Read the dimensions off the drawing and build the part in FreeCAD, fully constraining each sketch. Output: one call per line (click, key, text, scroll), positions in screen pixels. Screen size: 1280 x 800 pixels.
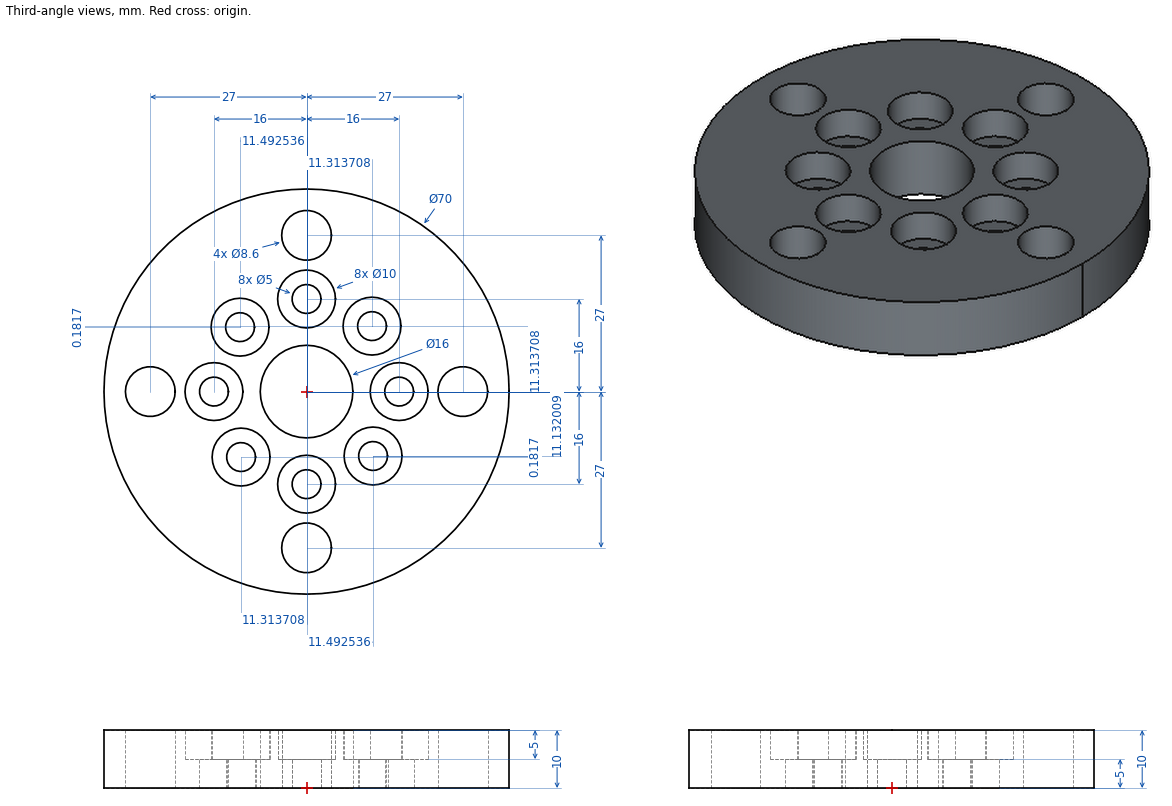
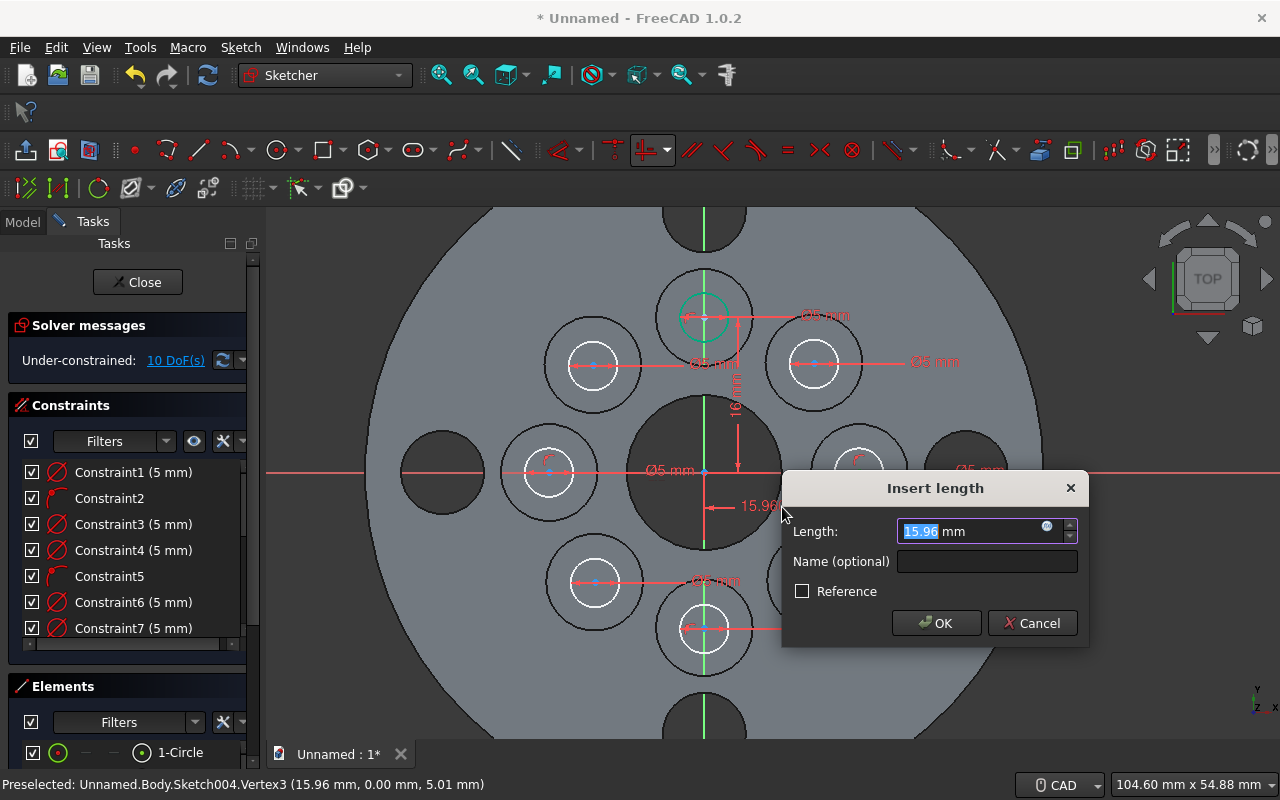
text(16)
key(Return)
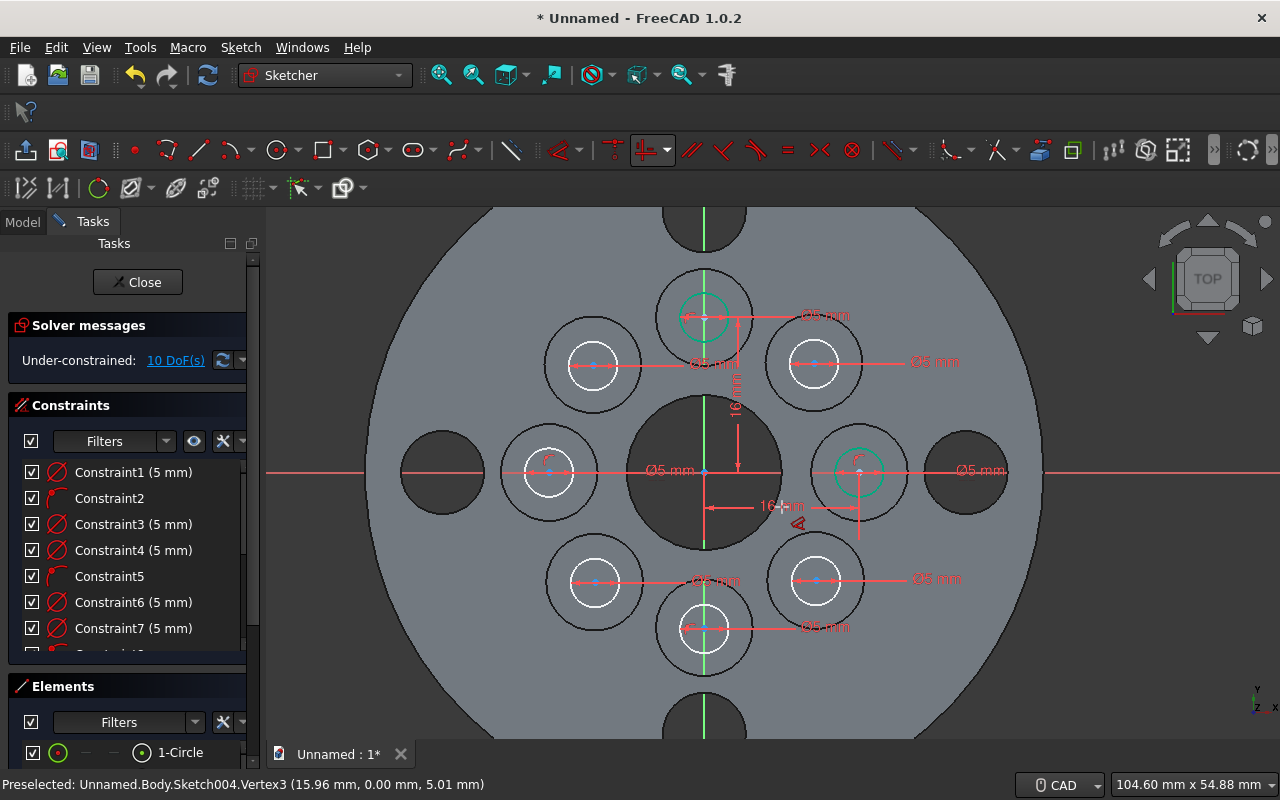
click(704, 629)
click(738, 551)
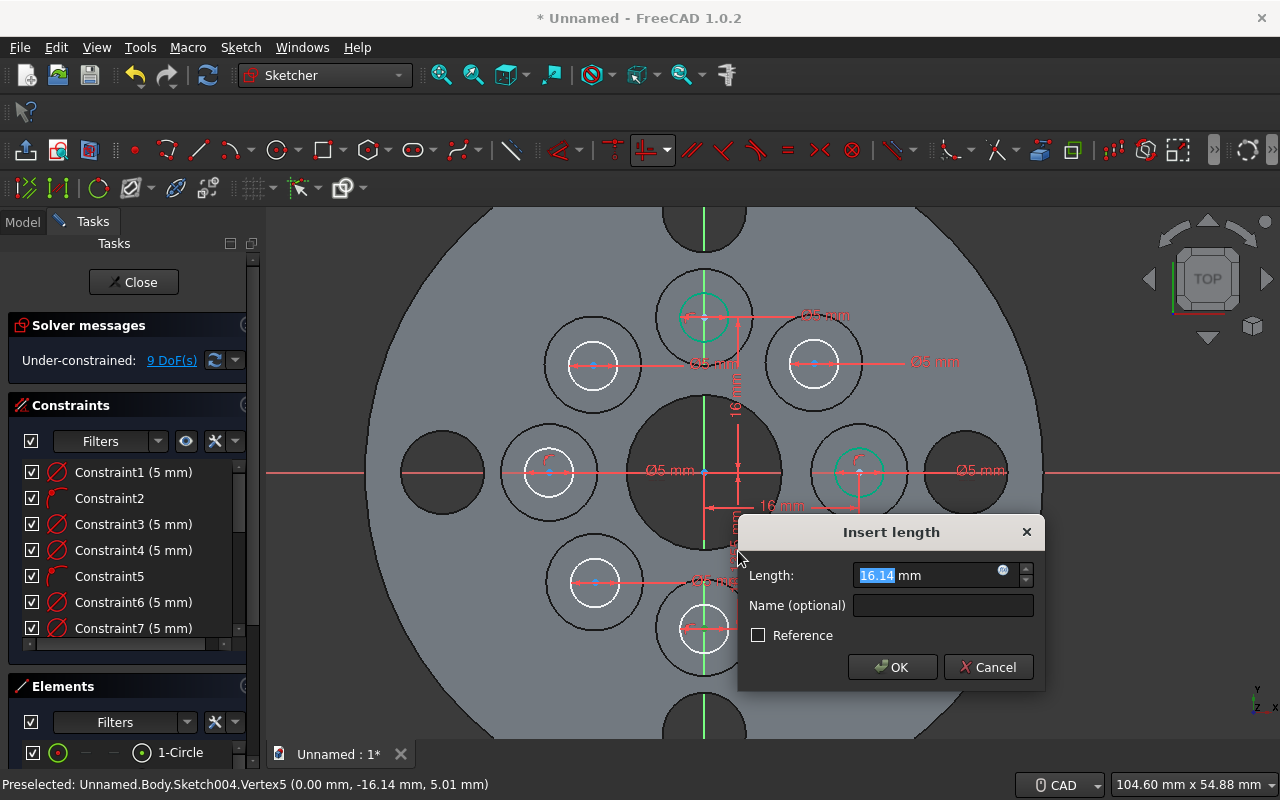
text(16)
key(Return)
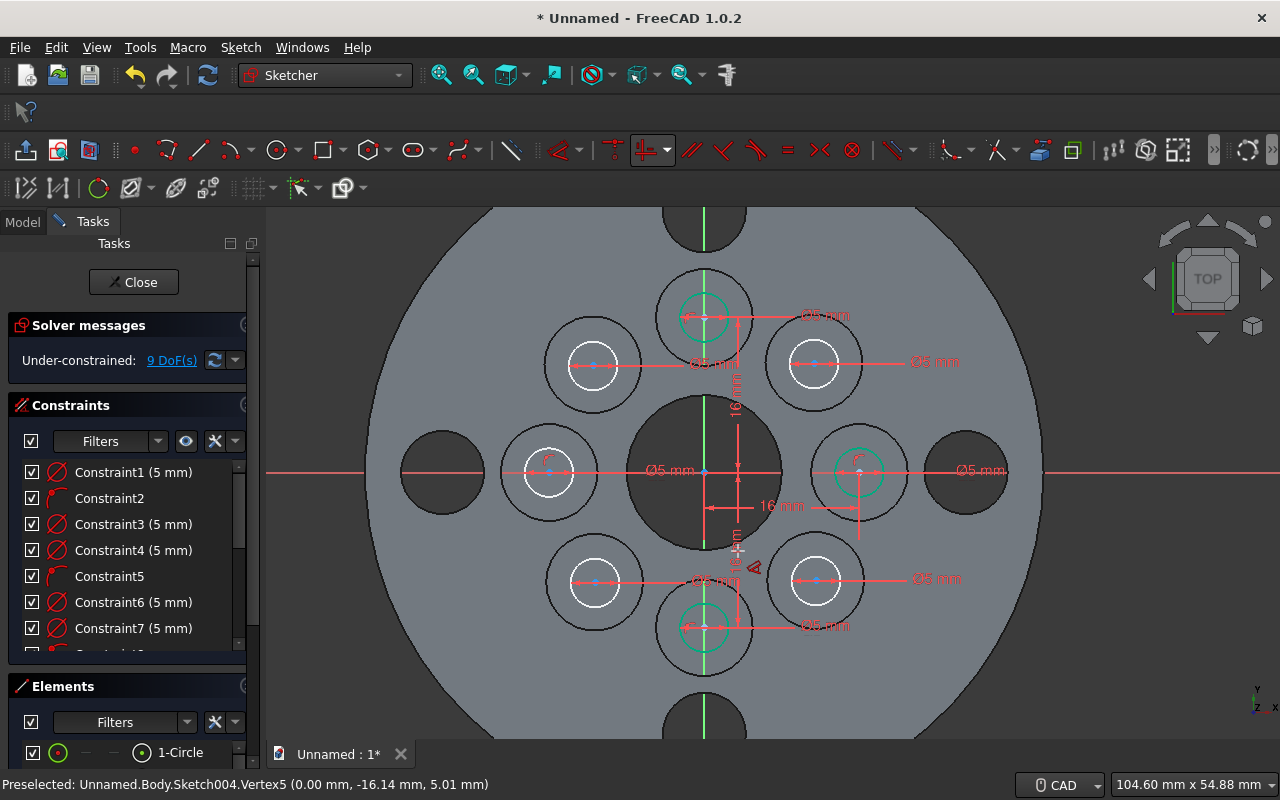
click(549, 473)
click(627, 507)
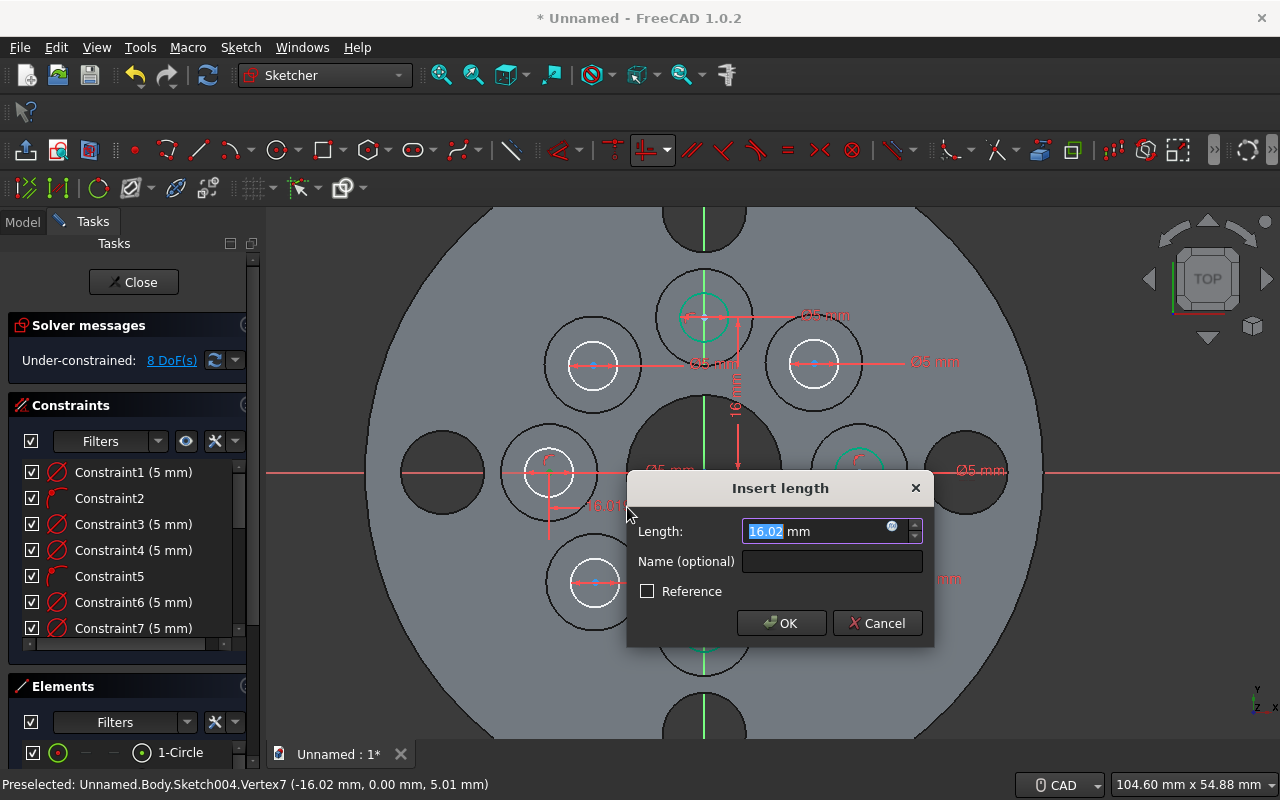
text(16)
key(Return)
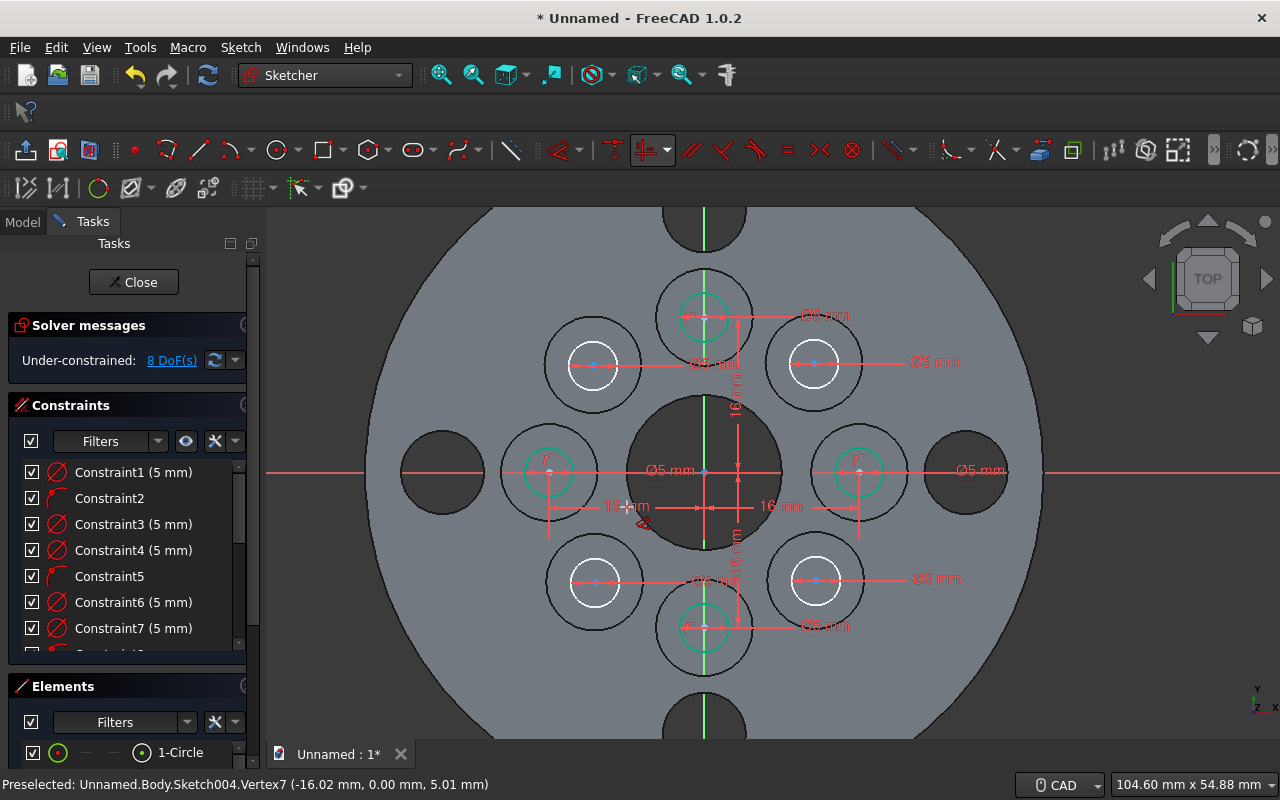
scroll(816, 581, up, 16)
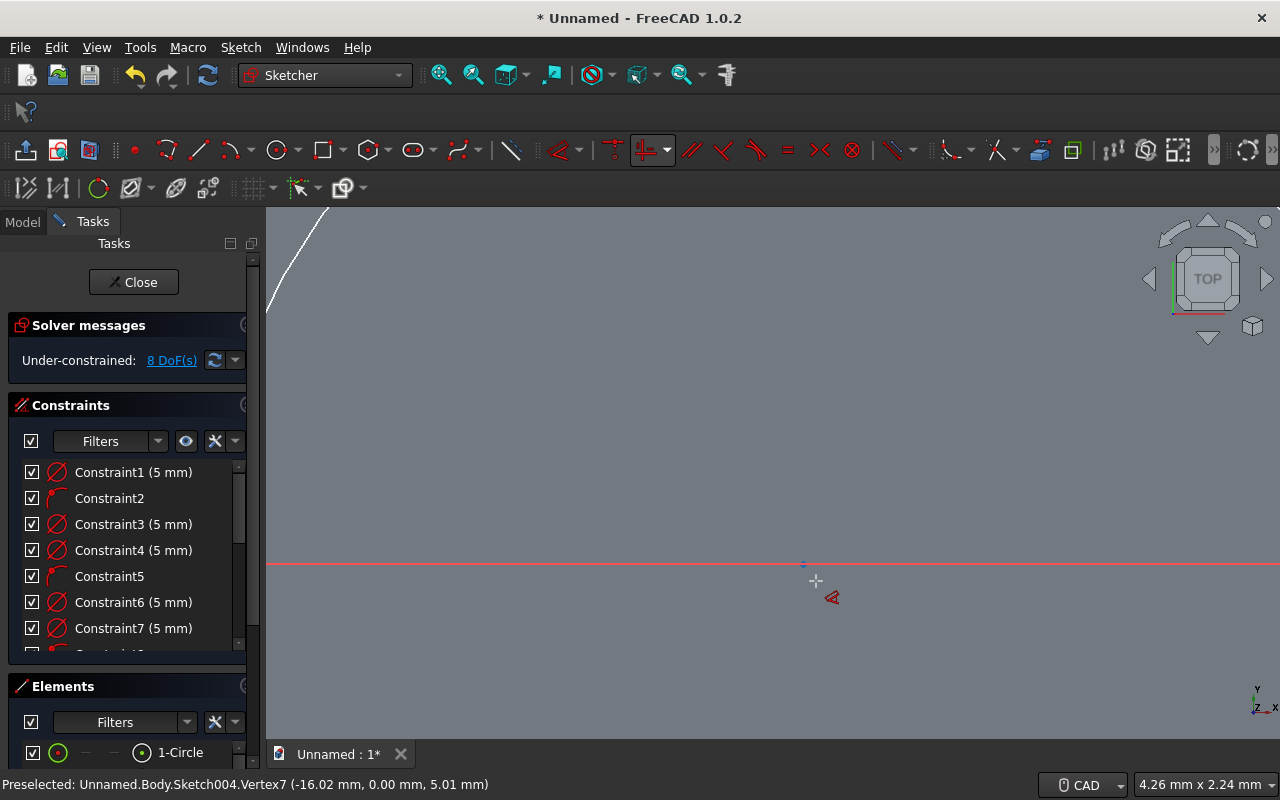
click(803, 564)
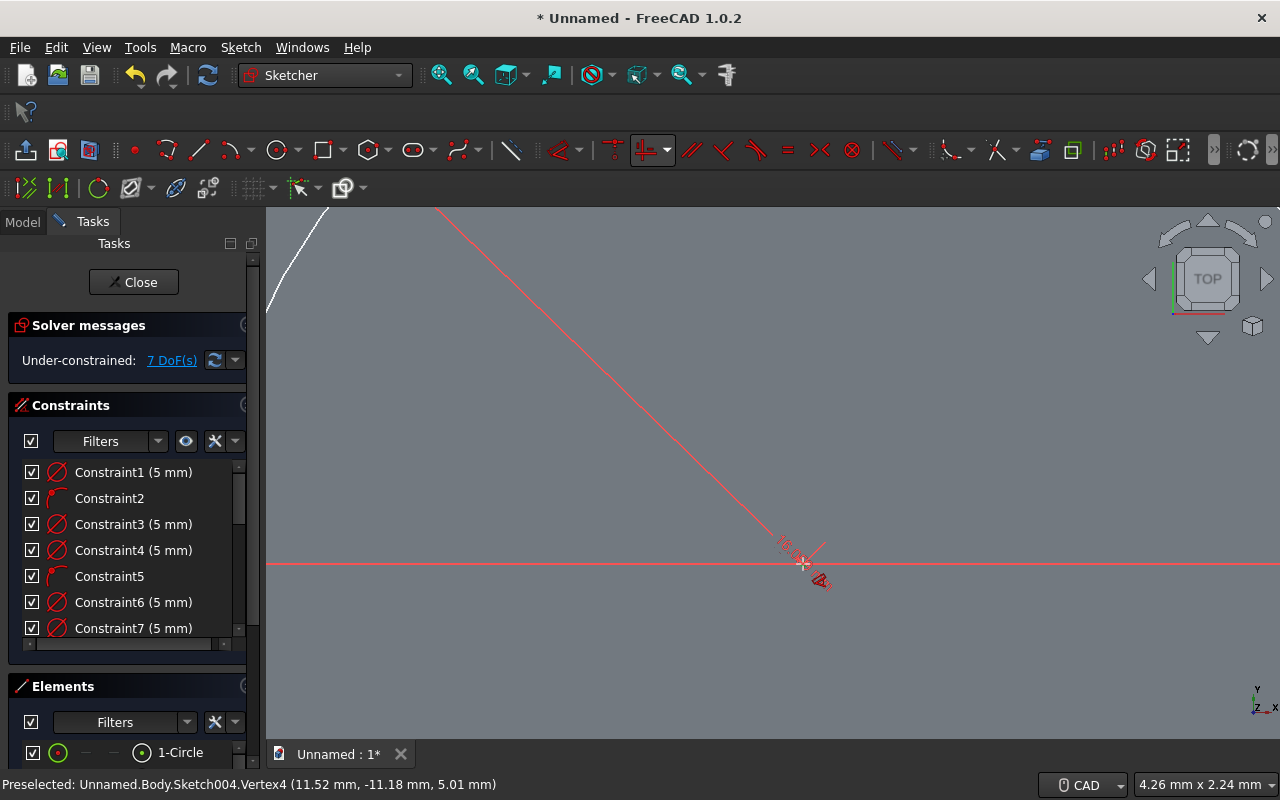
scroll(817, 582, down, 16)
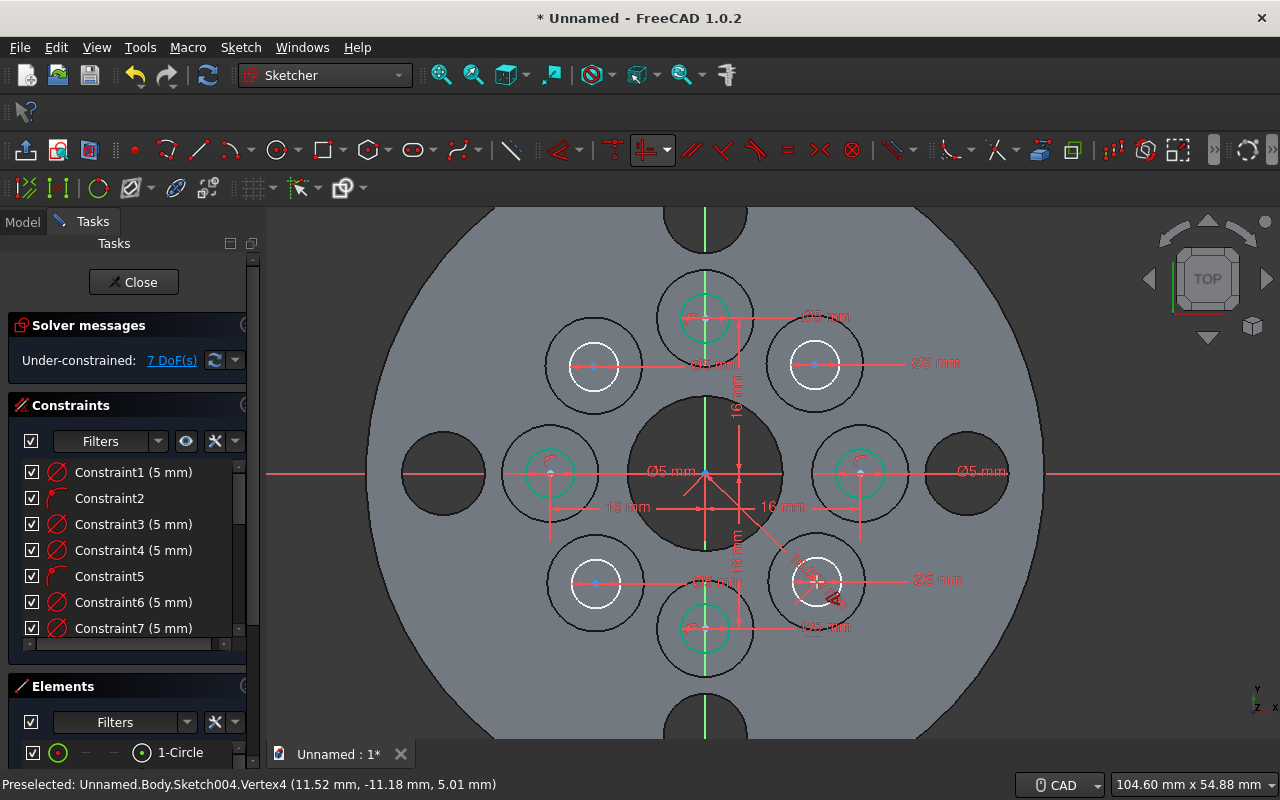
scroll(596, 584, up, 16)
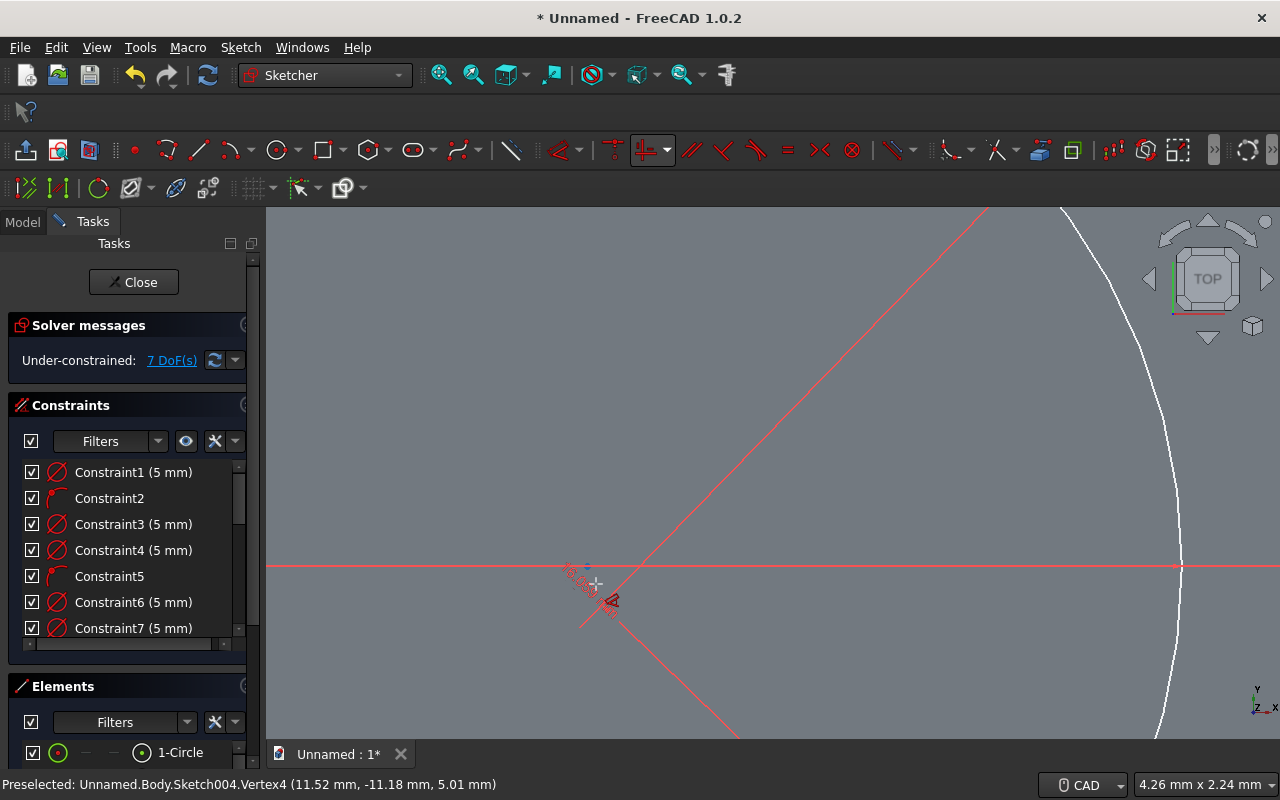
click(587, 566)
click(553, 542)